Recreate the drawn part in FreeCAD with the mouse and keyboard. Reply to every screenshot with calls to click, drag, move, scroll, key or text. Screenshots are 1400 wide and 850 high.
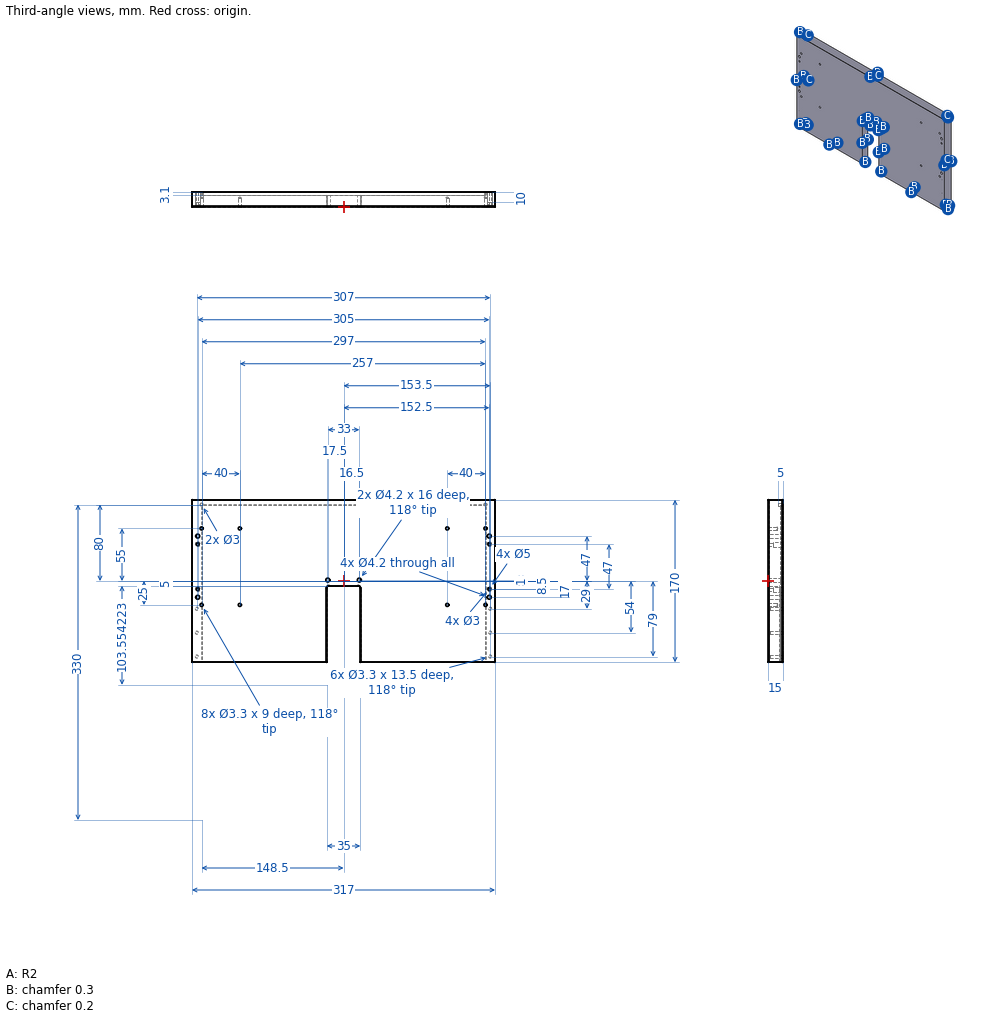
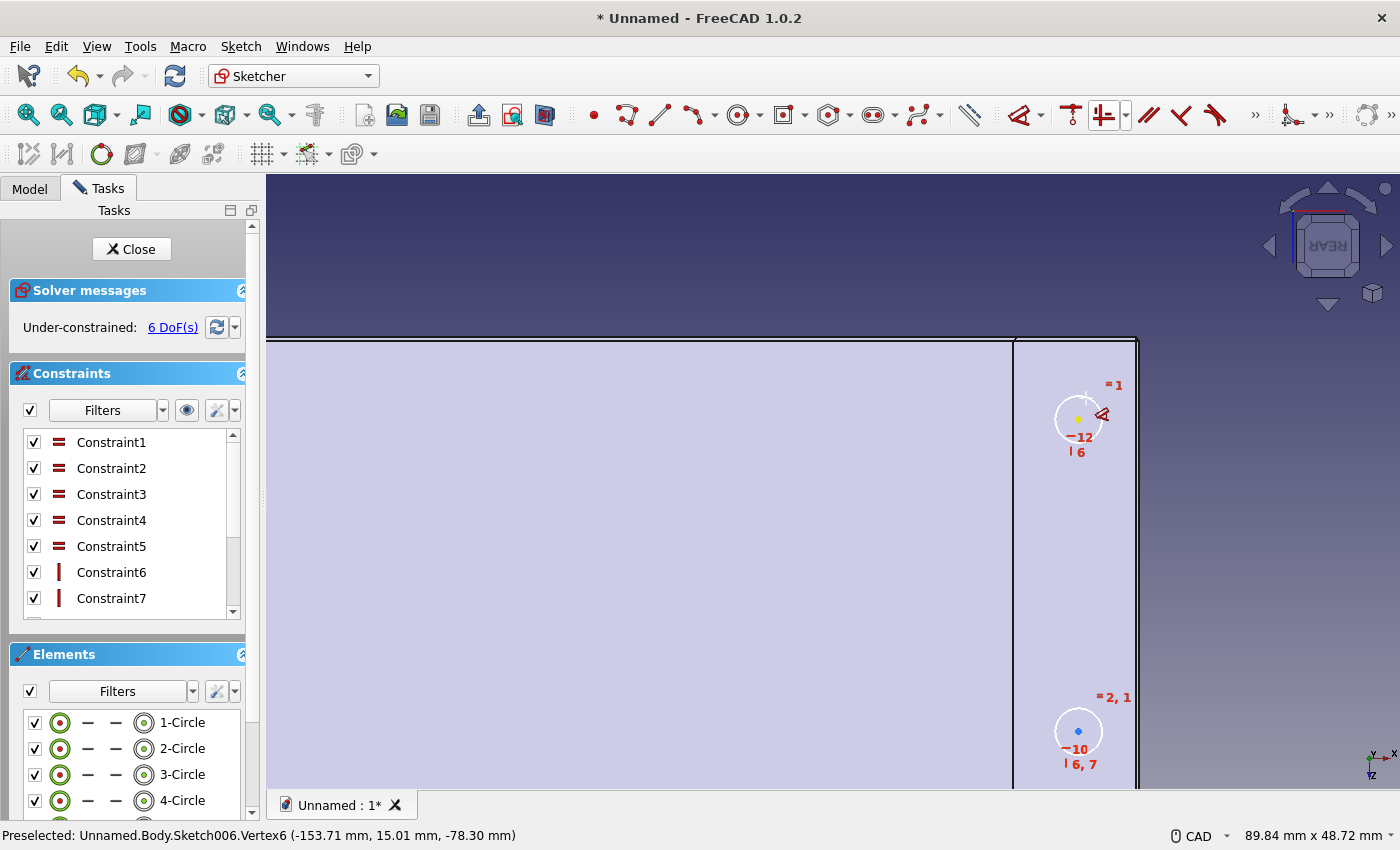
click(1079, 396)
click(1079, 364)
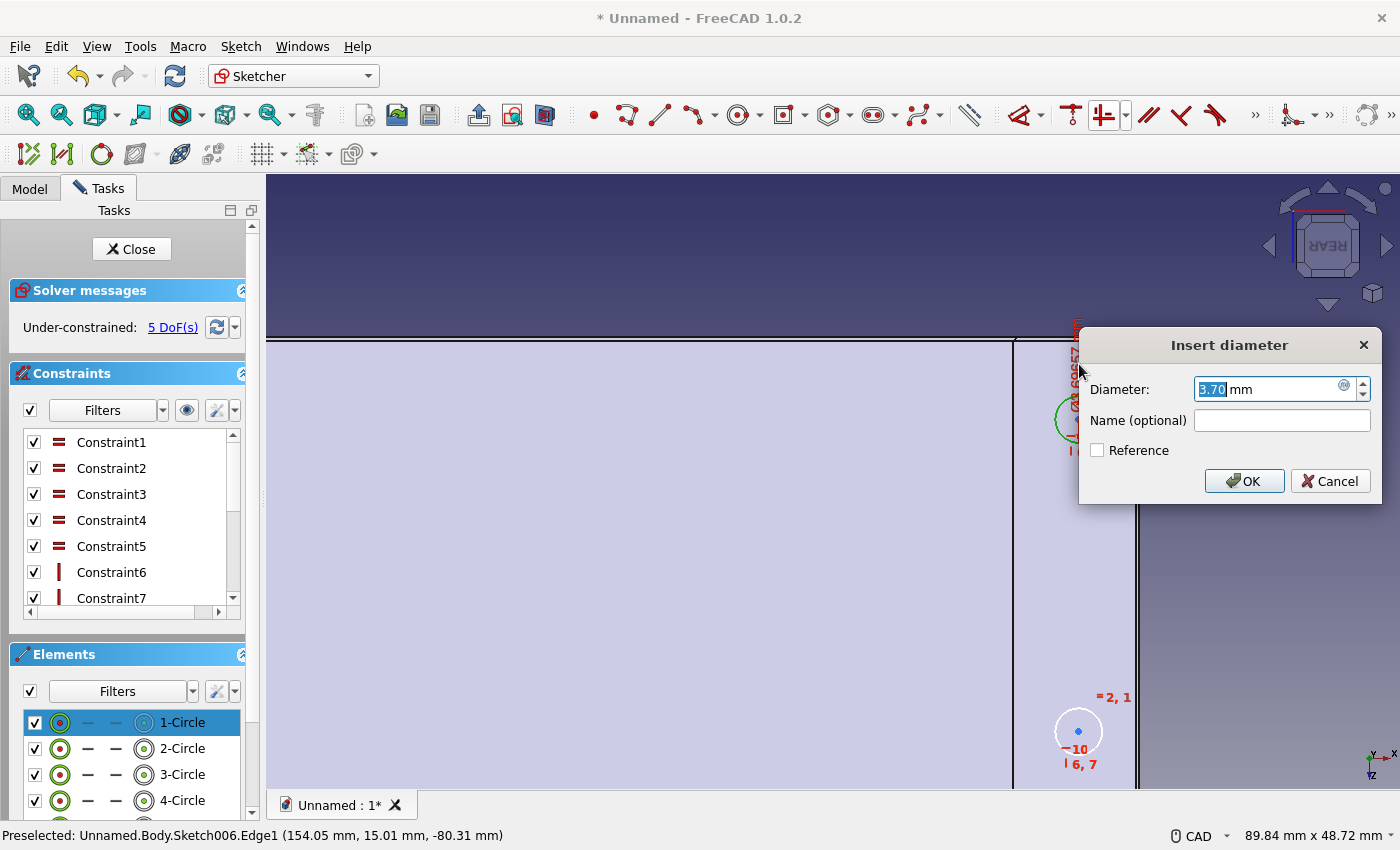
text(3.3)
key(Return)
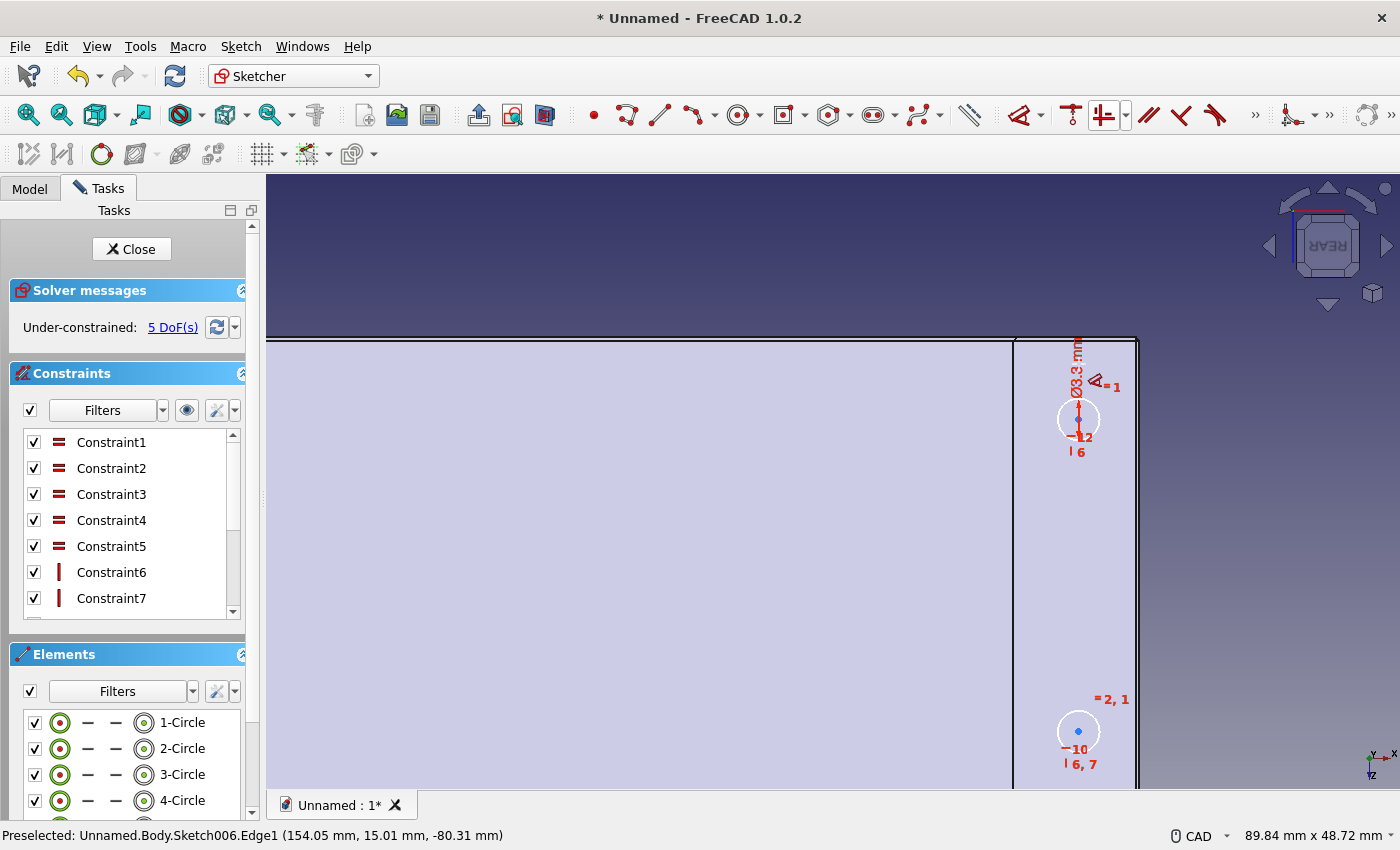
scroll(1086, 398, down, 9)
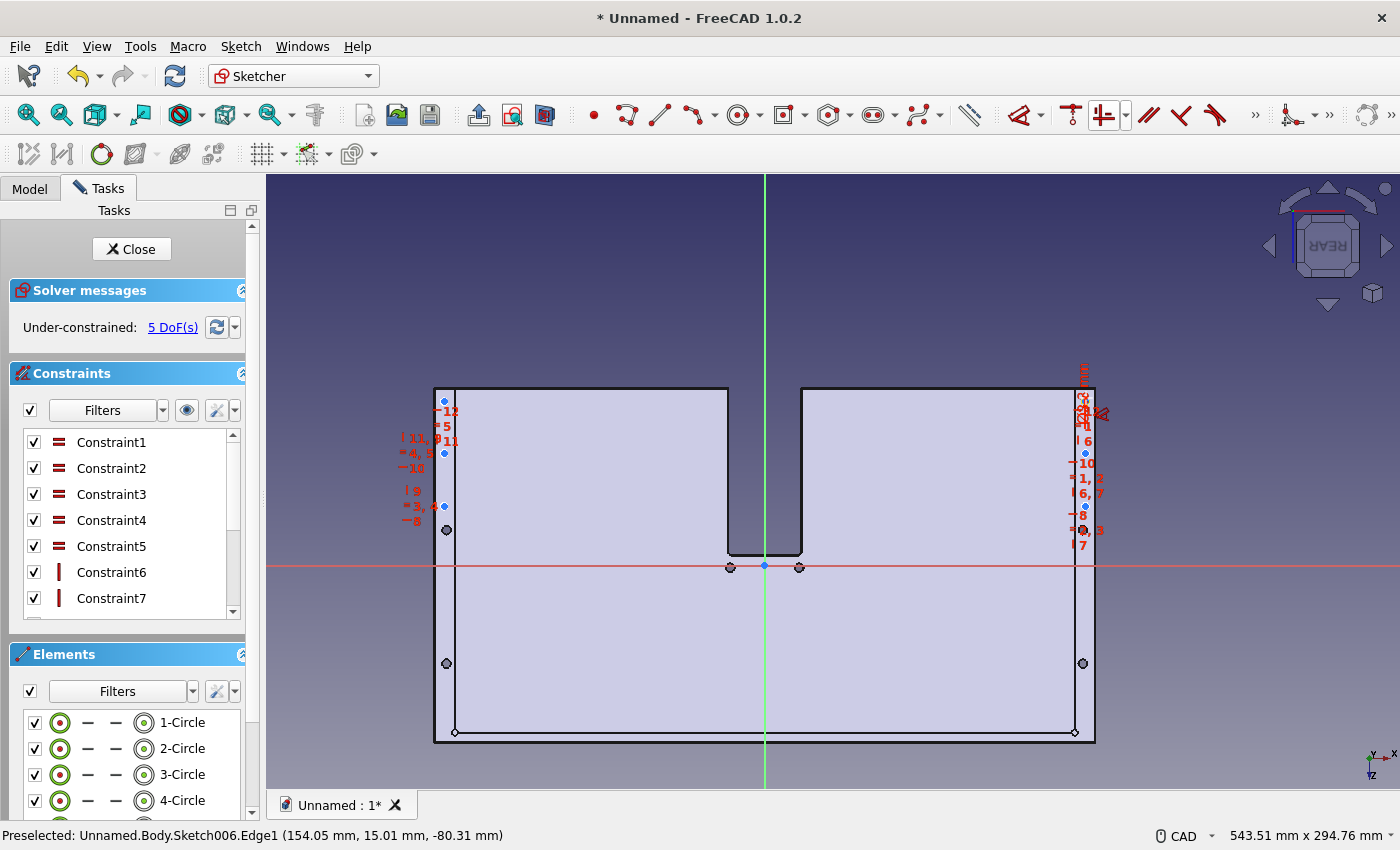
click(1085, 402)
click(1119, 484)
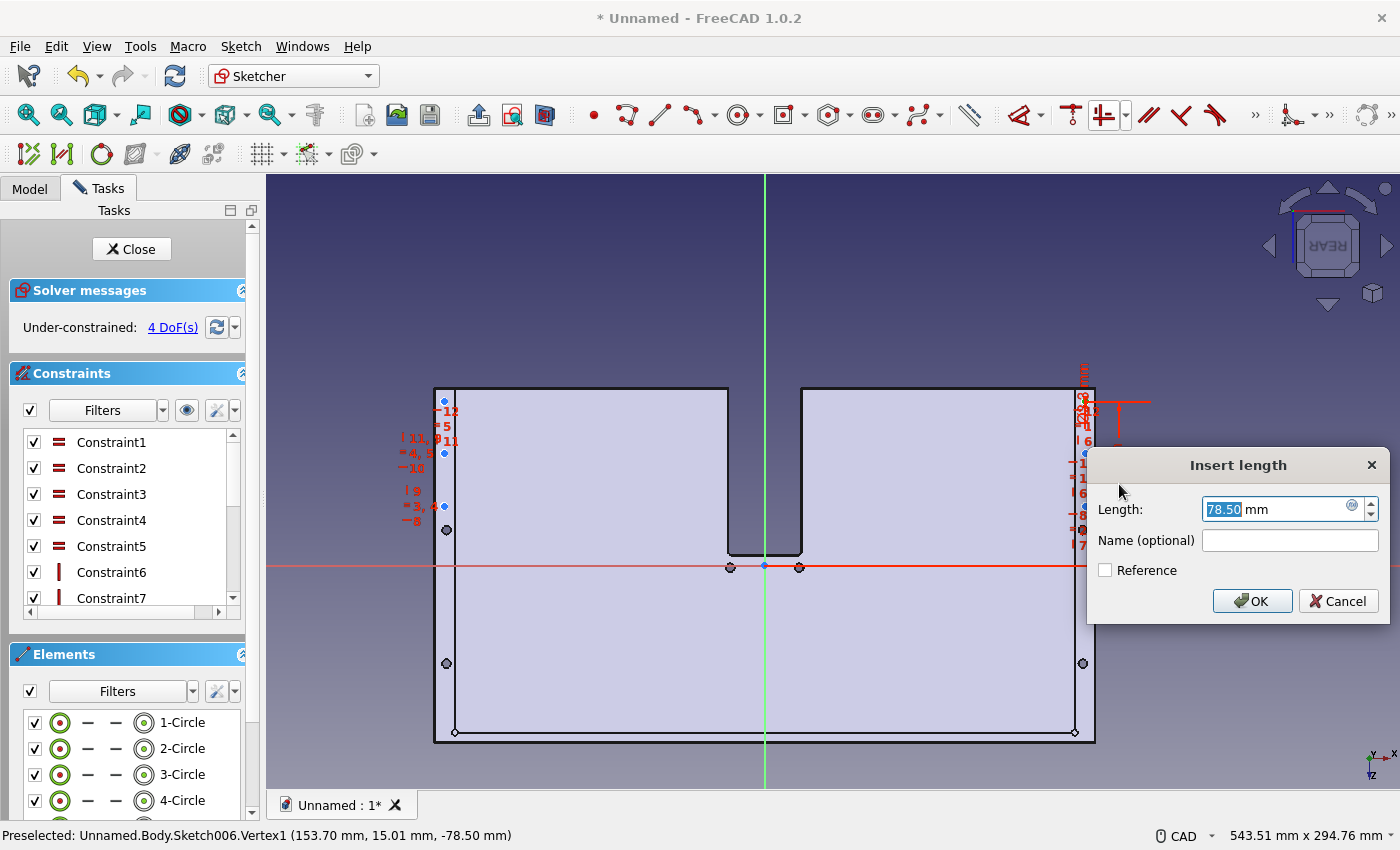
text(79)
key(Return)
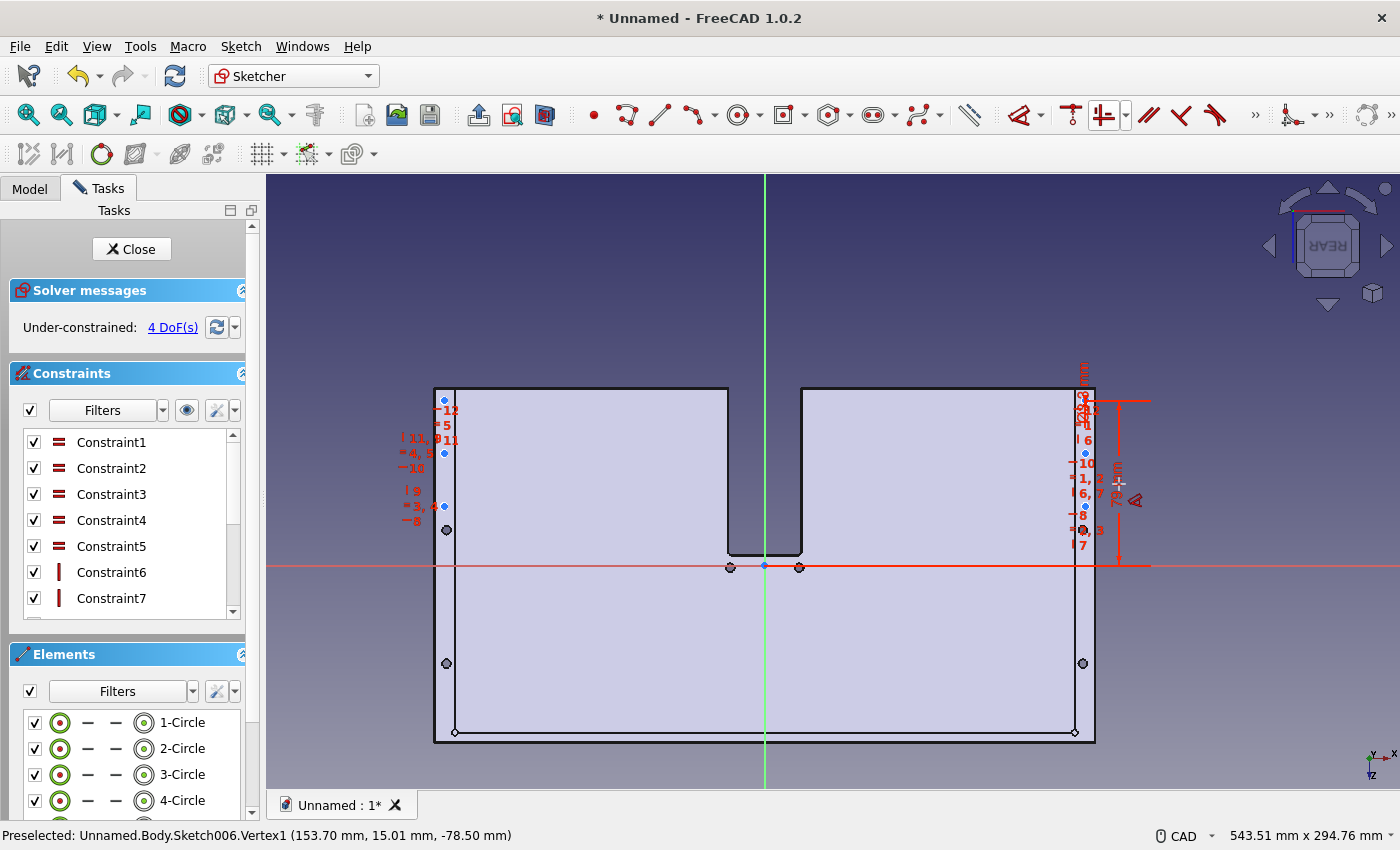
click(1085, 453)
click(1119, 510)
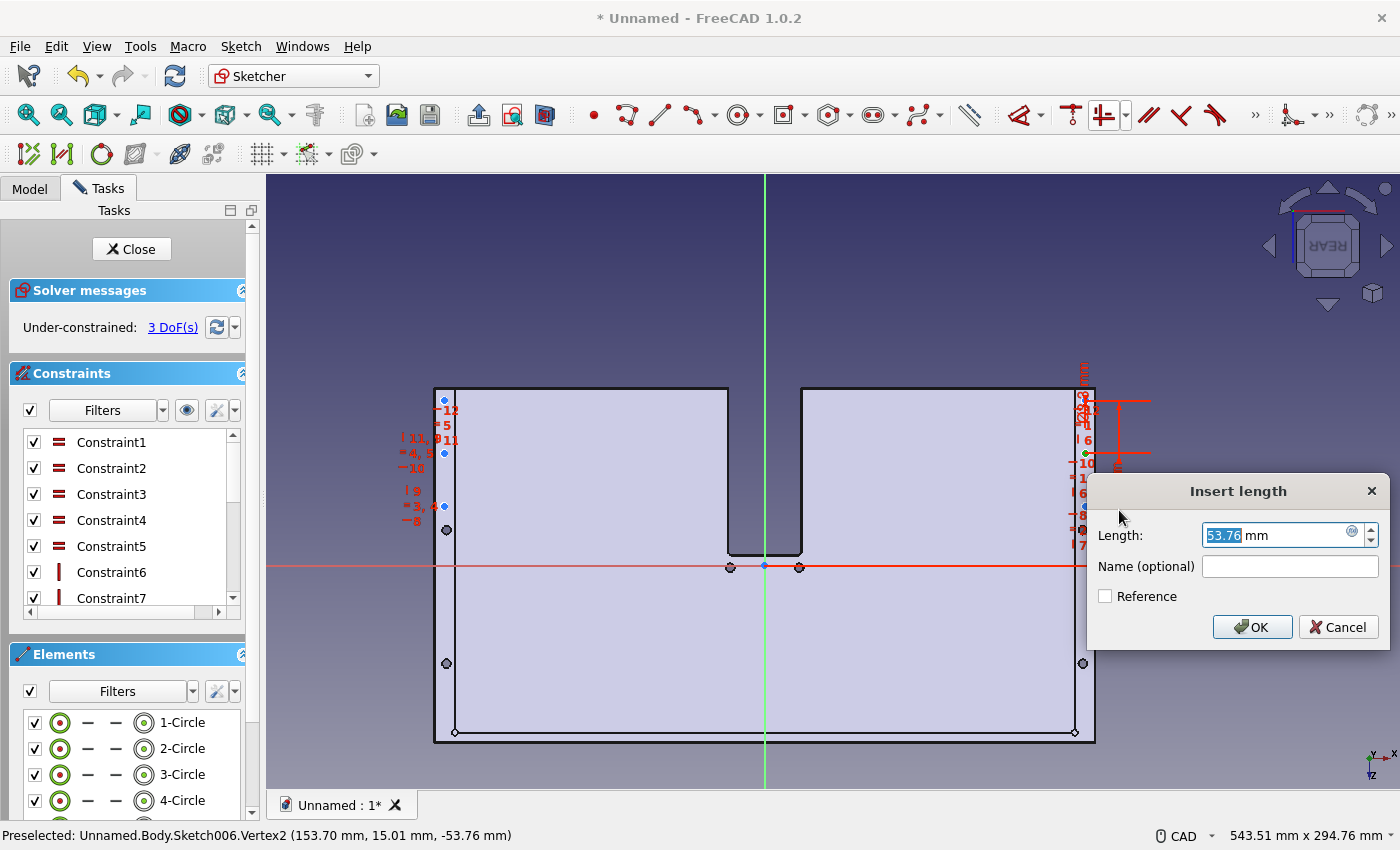
text(54)
key(Return)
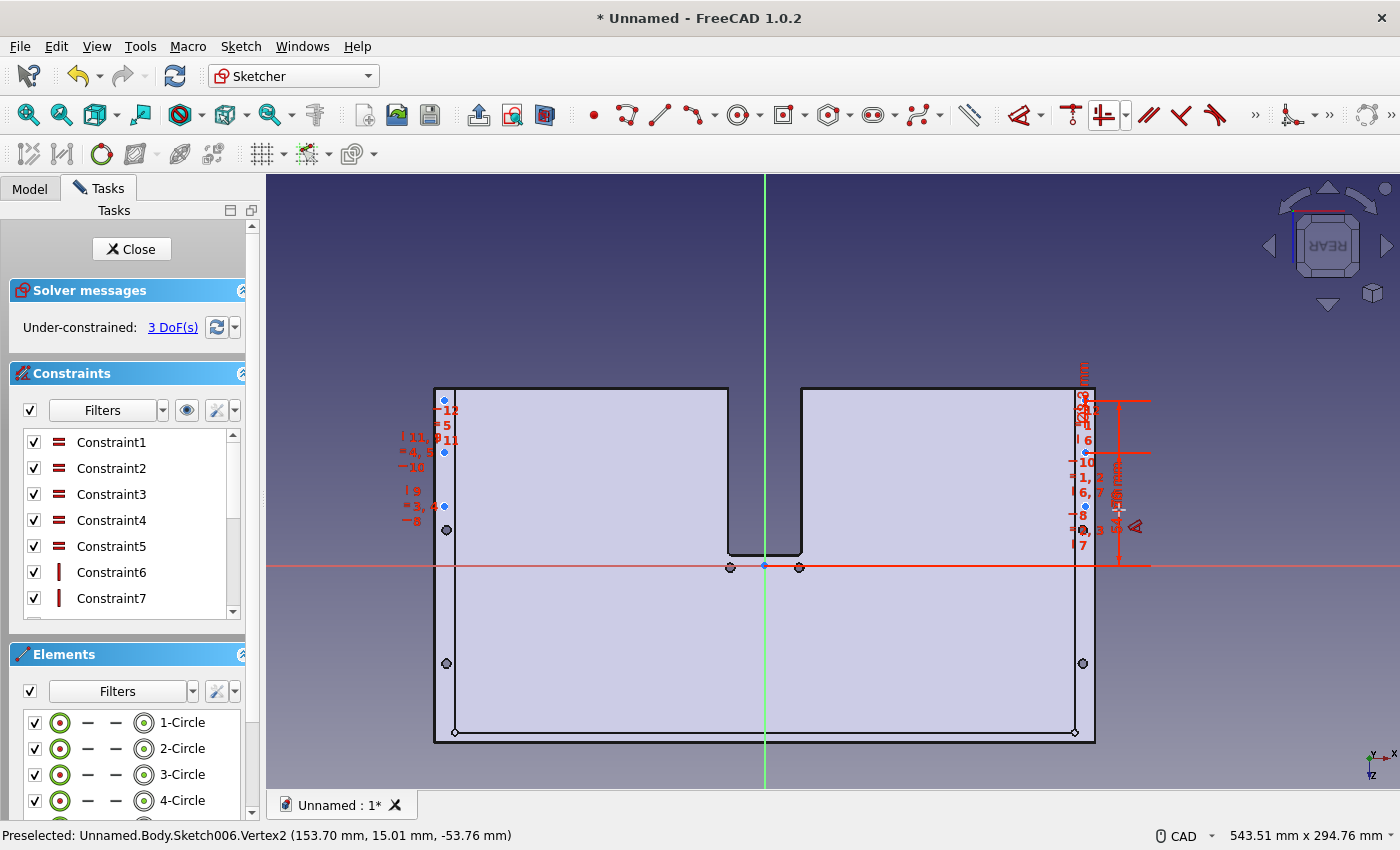
click(1085, 506)
click(1119, 536)